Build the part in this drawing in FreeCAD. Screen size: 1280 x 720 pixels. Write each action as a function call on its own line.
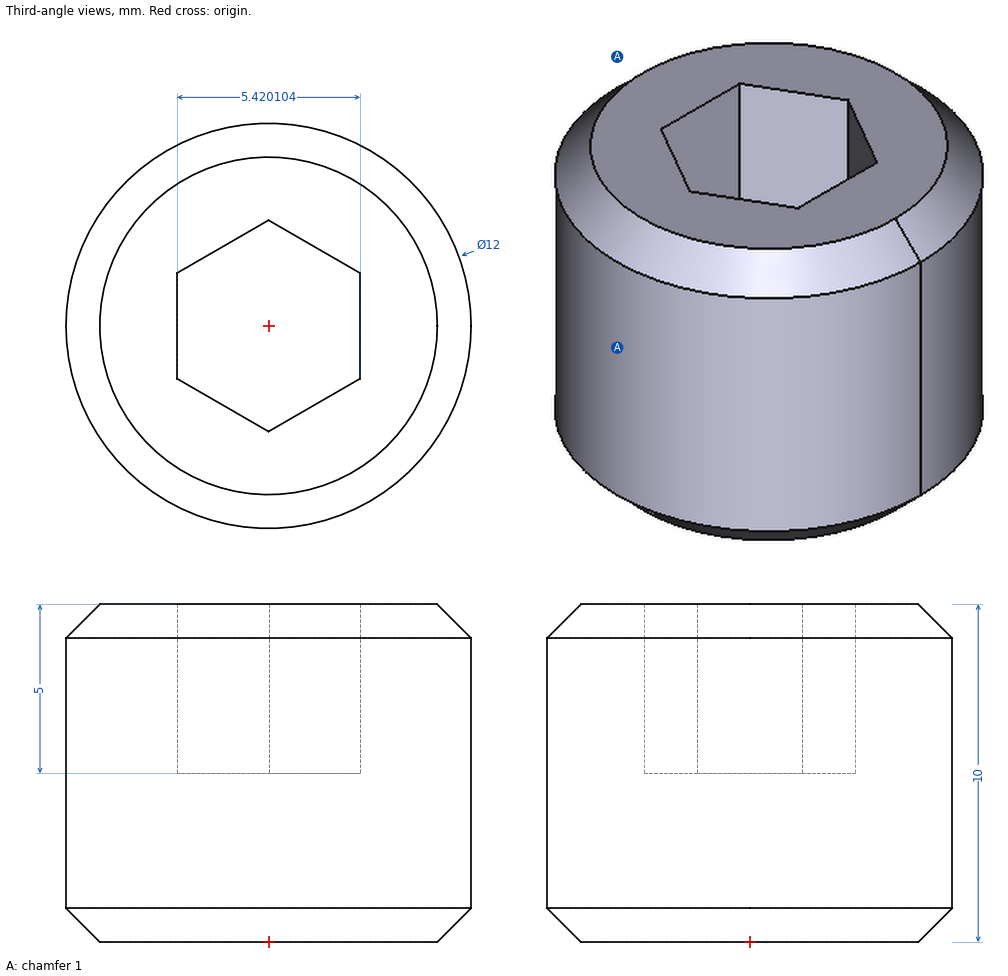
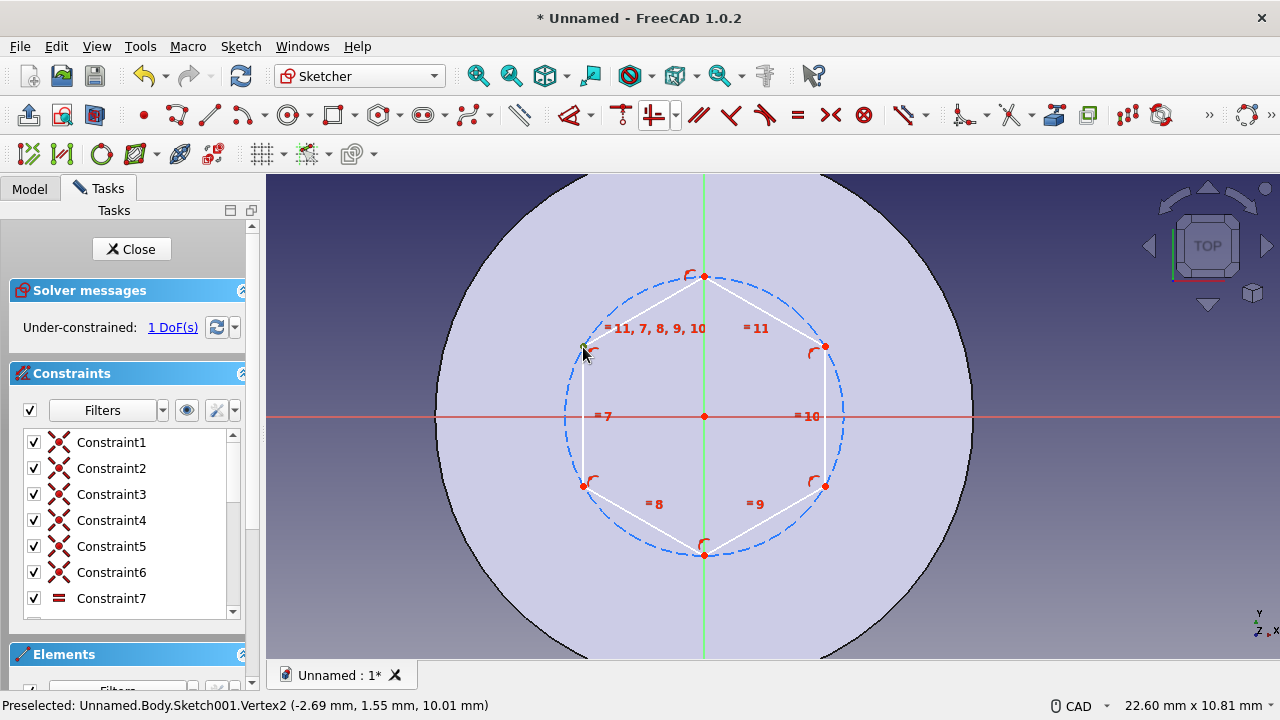
click(825, 486)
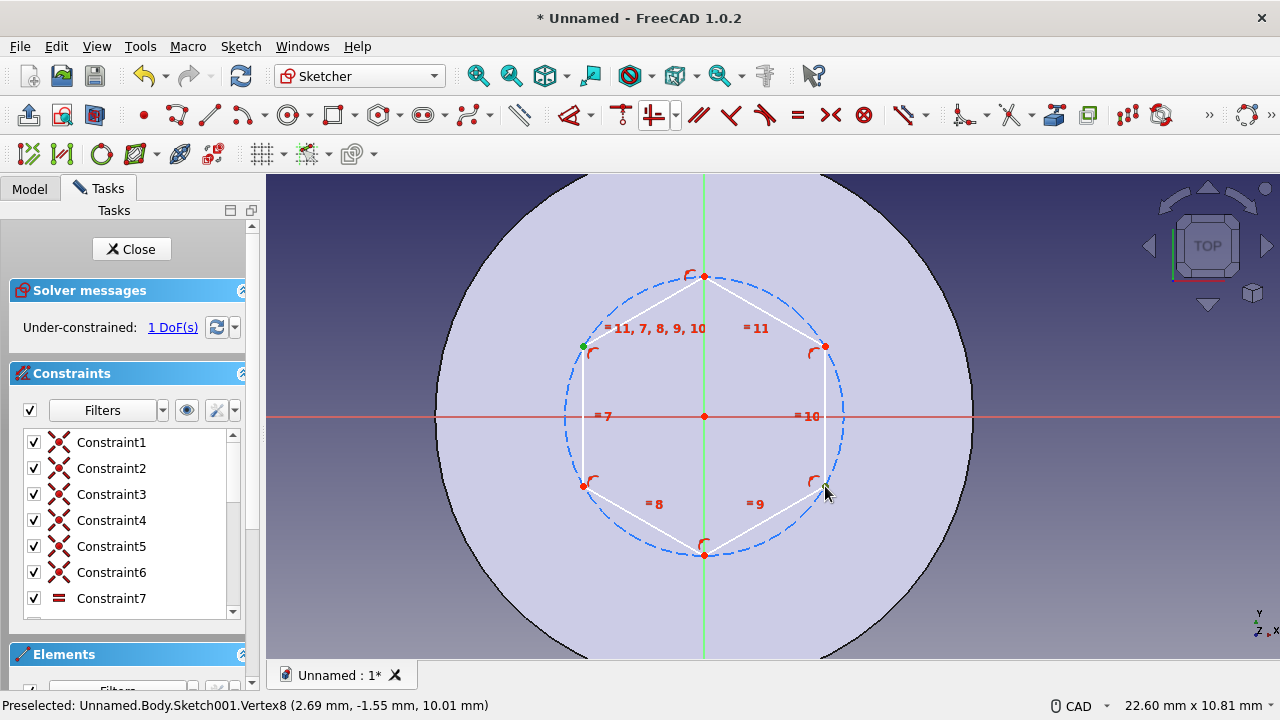
key(l)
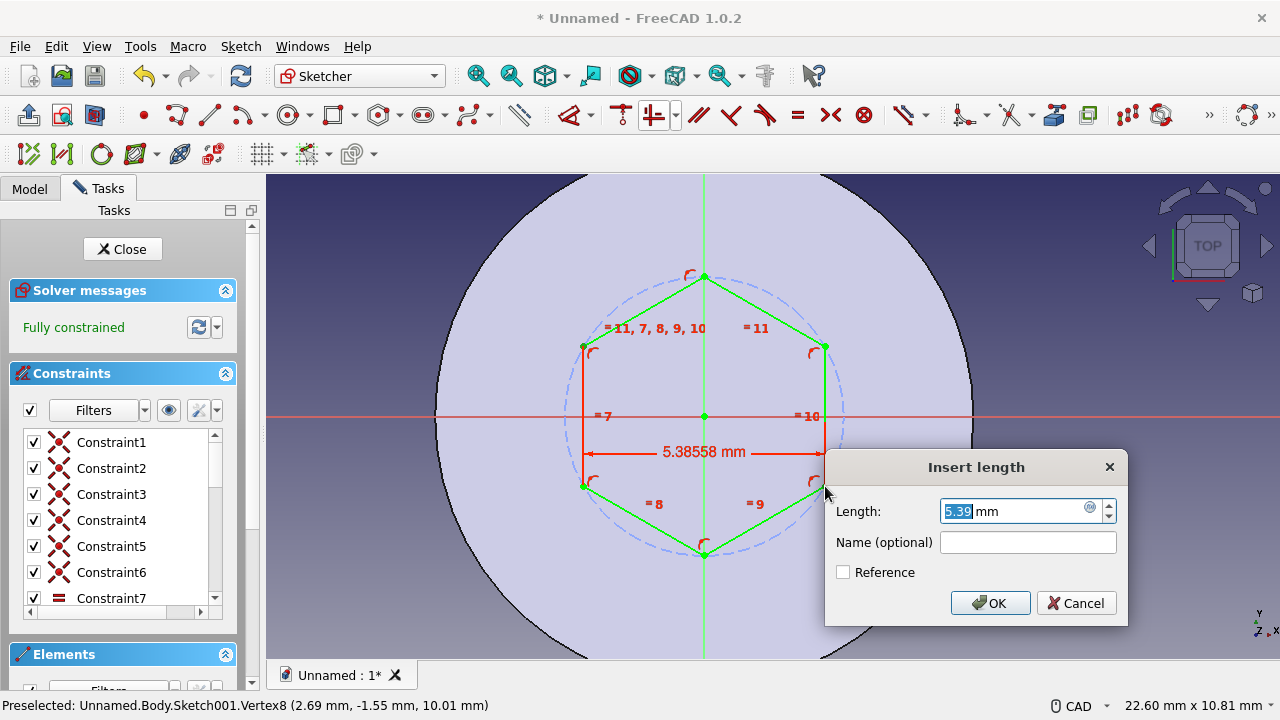
text(5.420104)
key(Return)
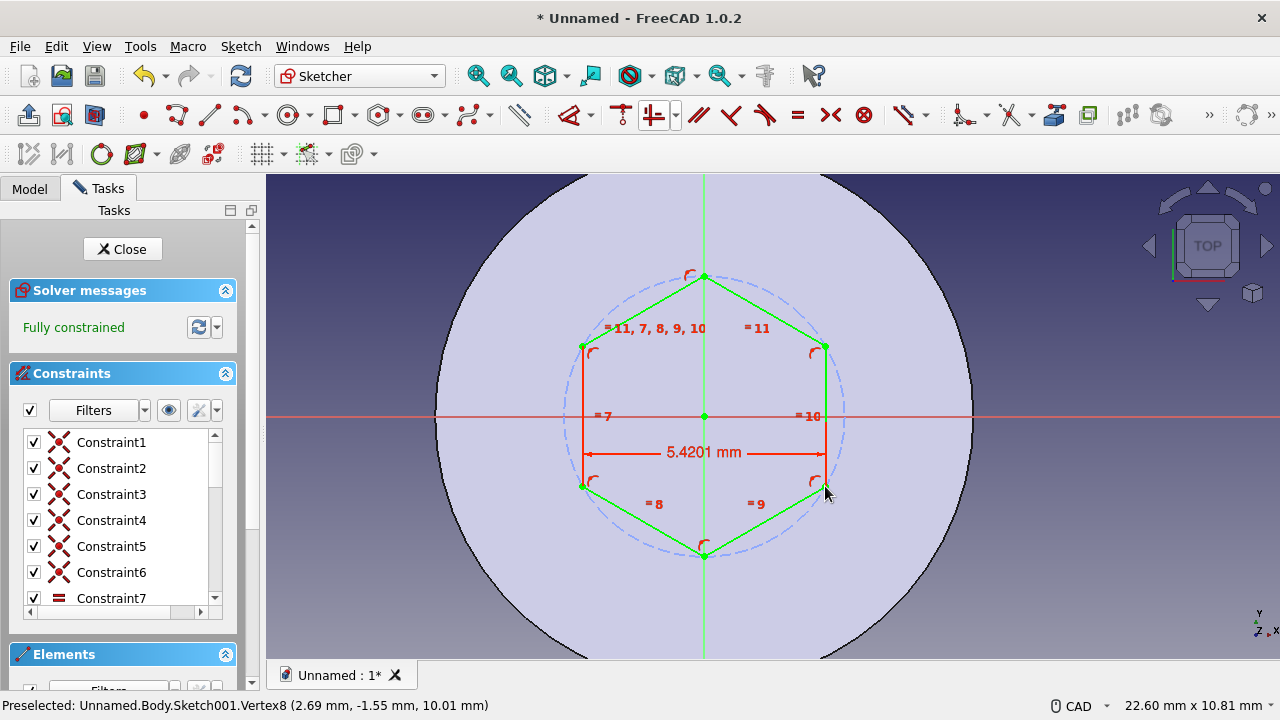
click(123, 249)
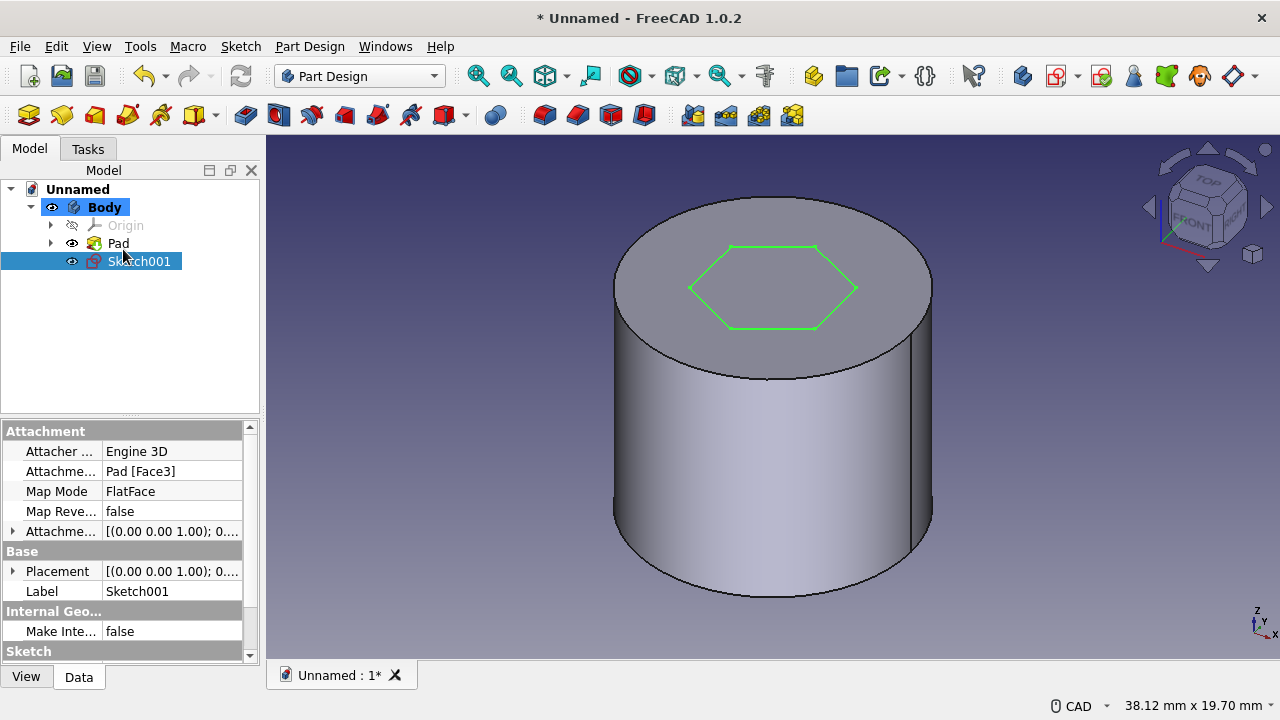
click(246, 116)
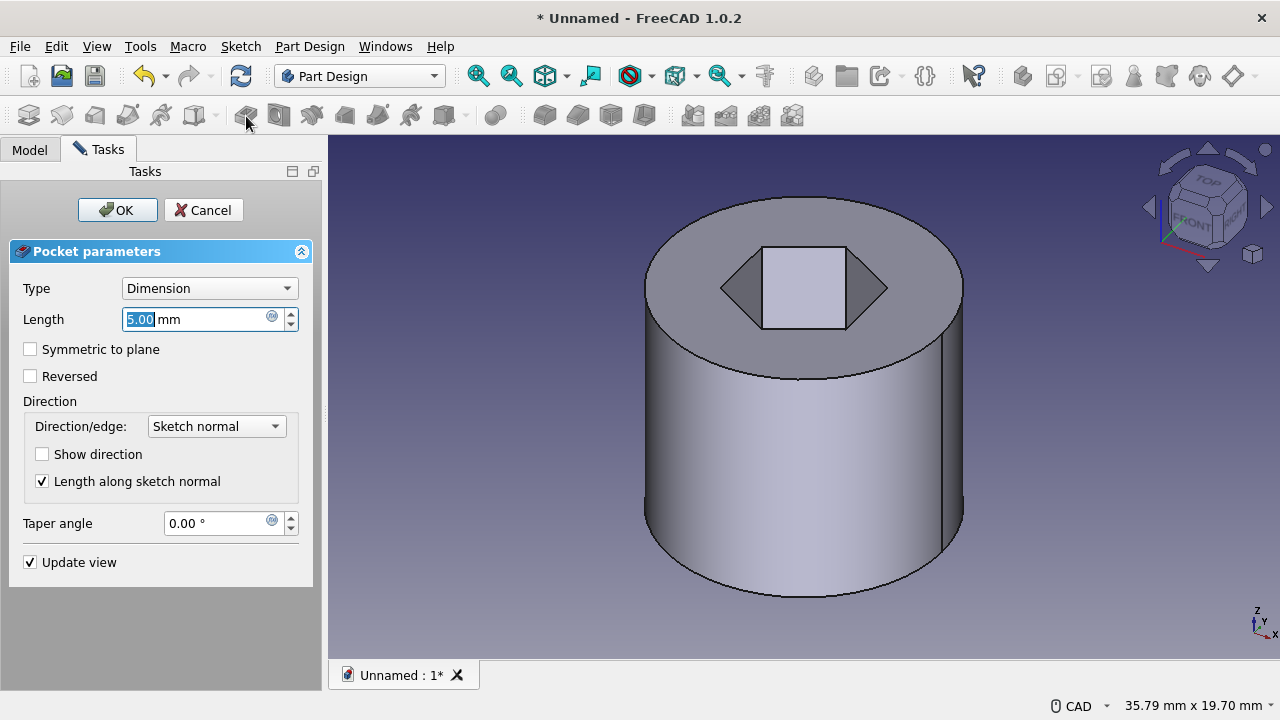
text(5)
key(Tab)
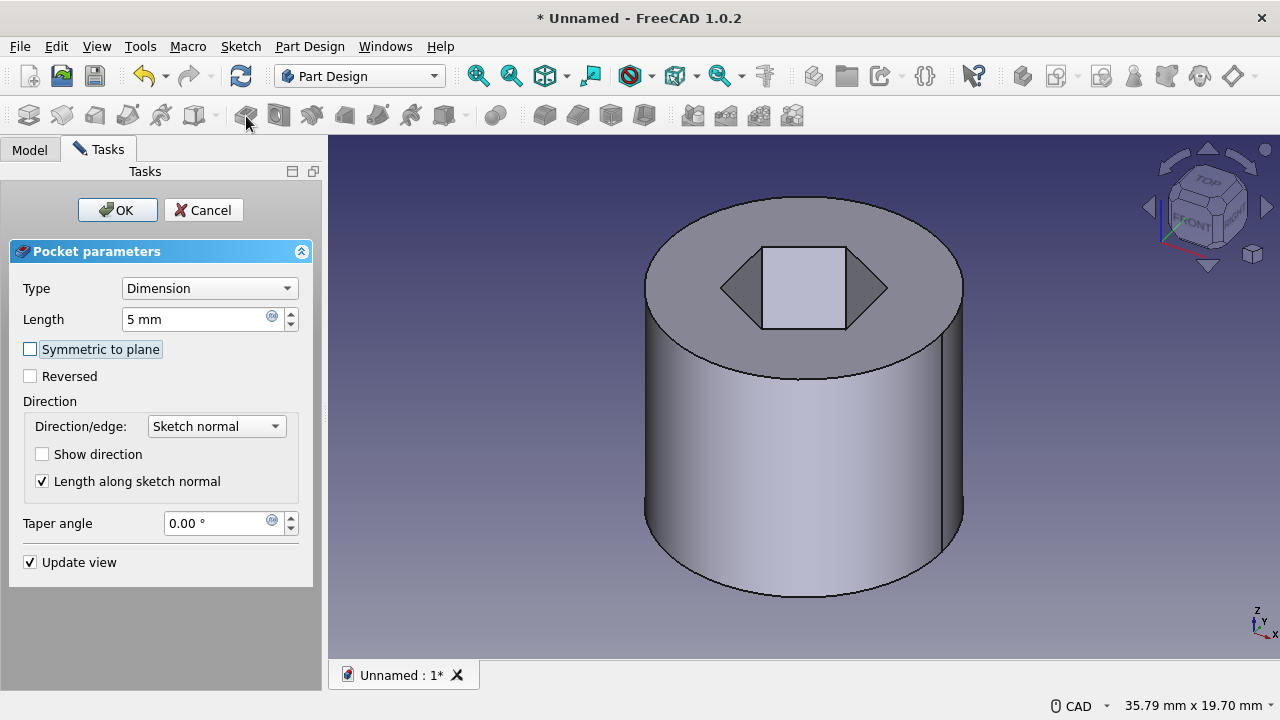
click(118, 210)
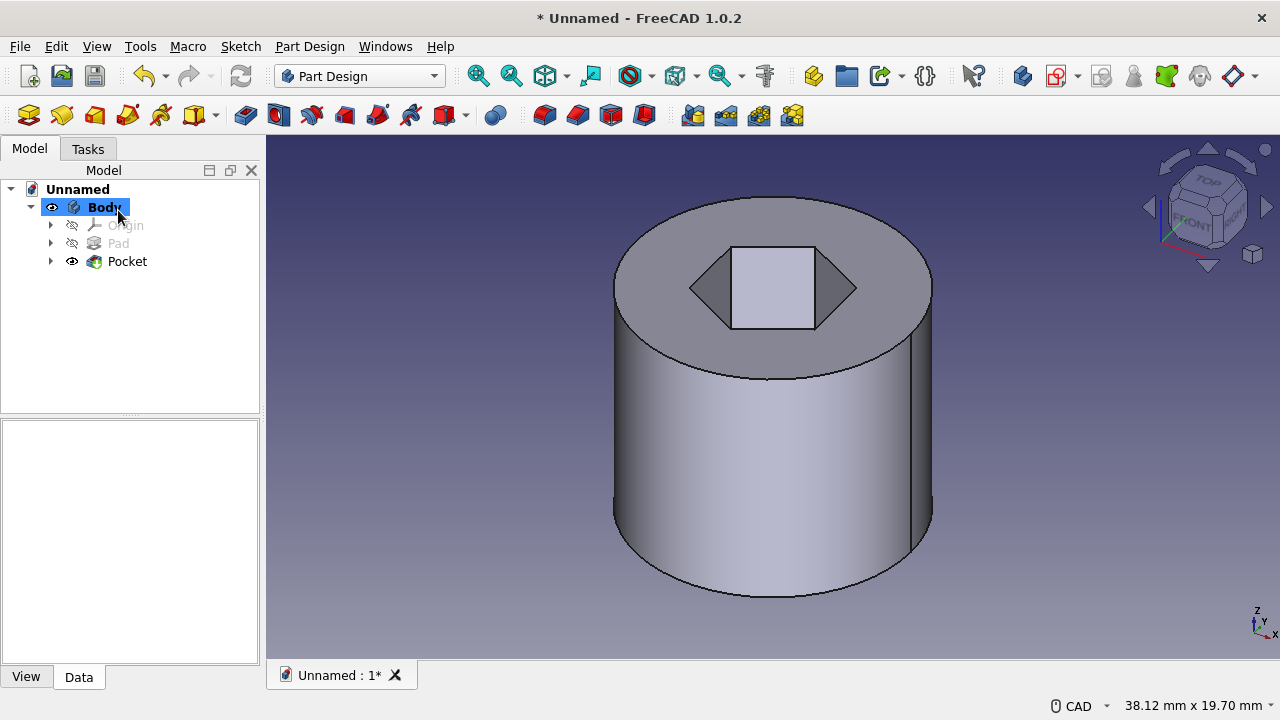
click(708, 203)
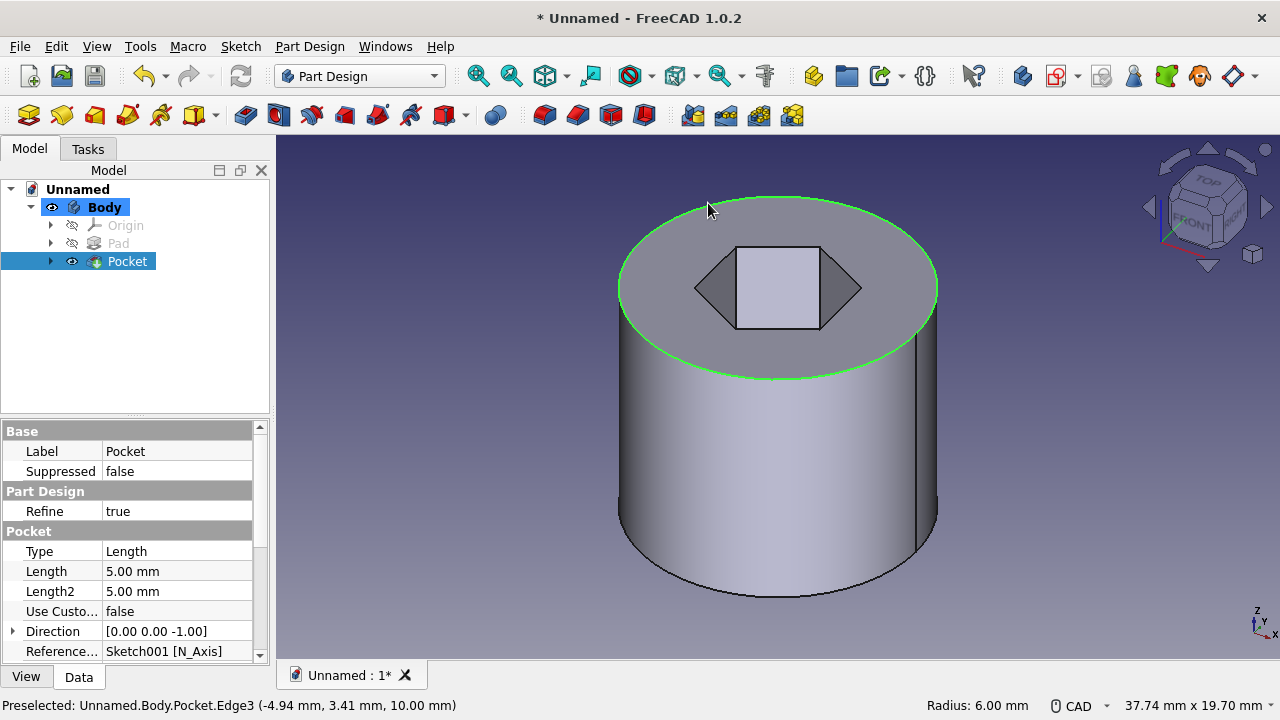
key(0)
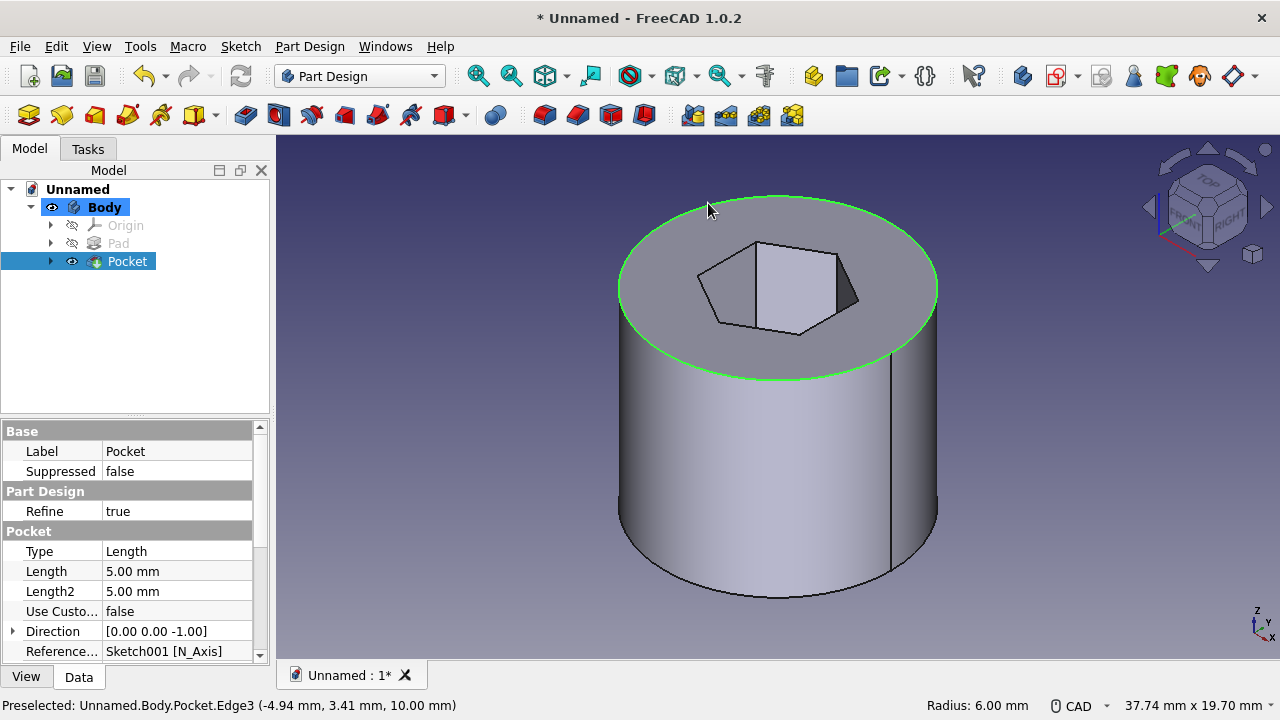
key(2)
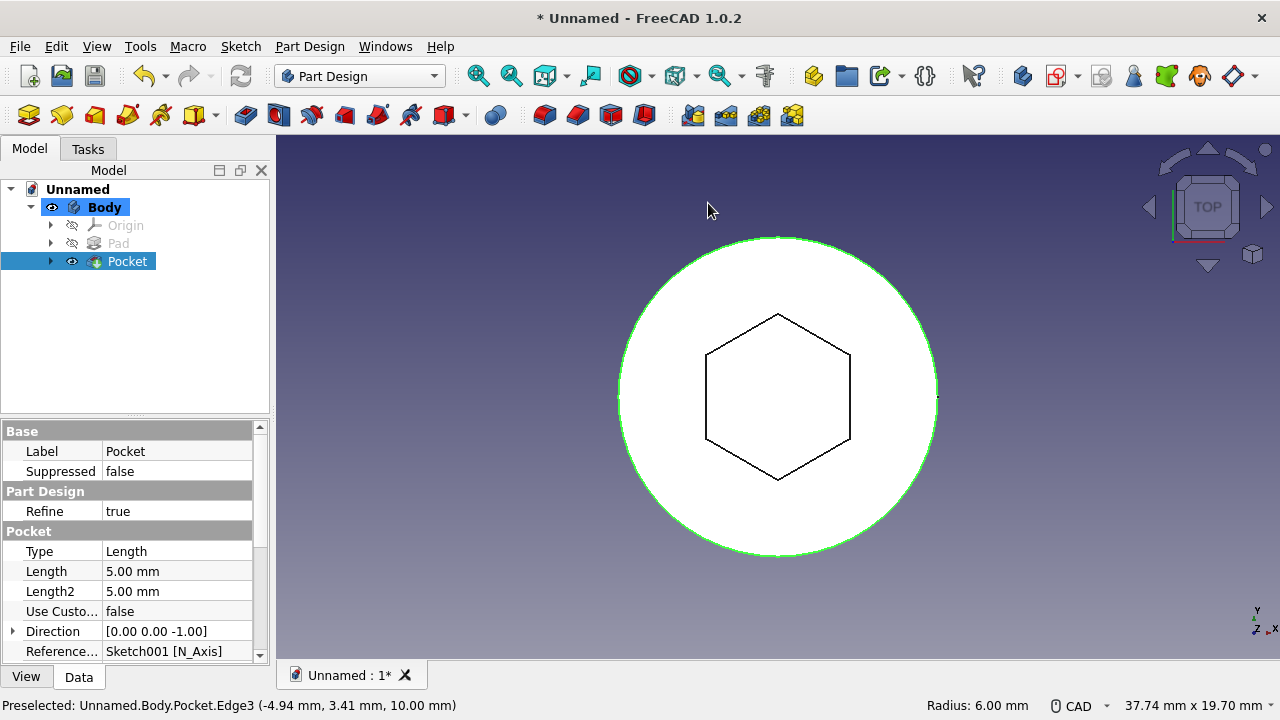
key(1)